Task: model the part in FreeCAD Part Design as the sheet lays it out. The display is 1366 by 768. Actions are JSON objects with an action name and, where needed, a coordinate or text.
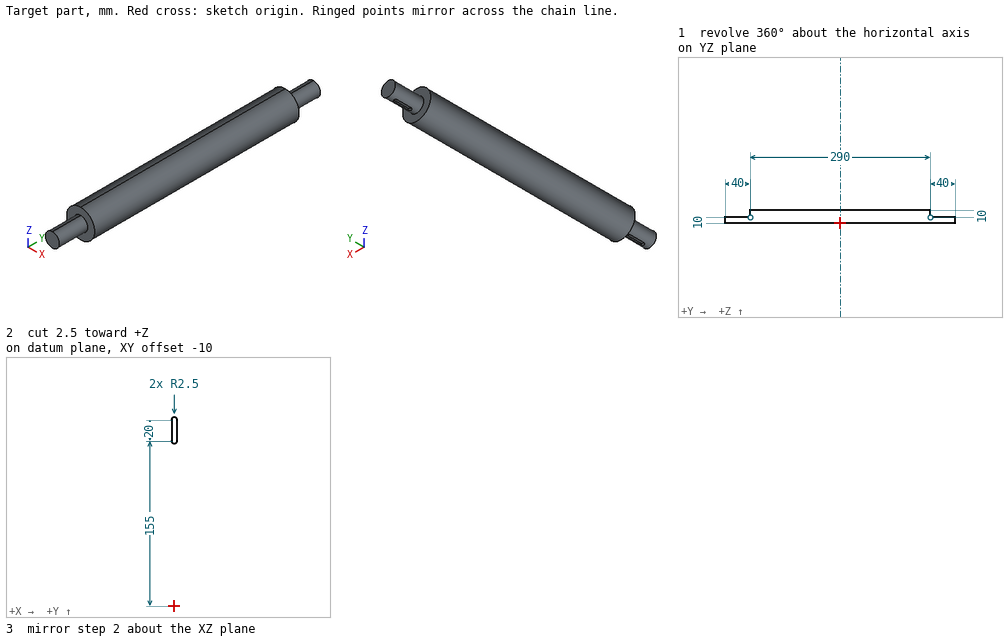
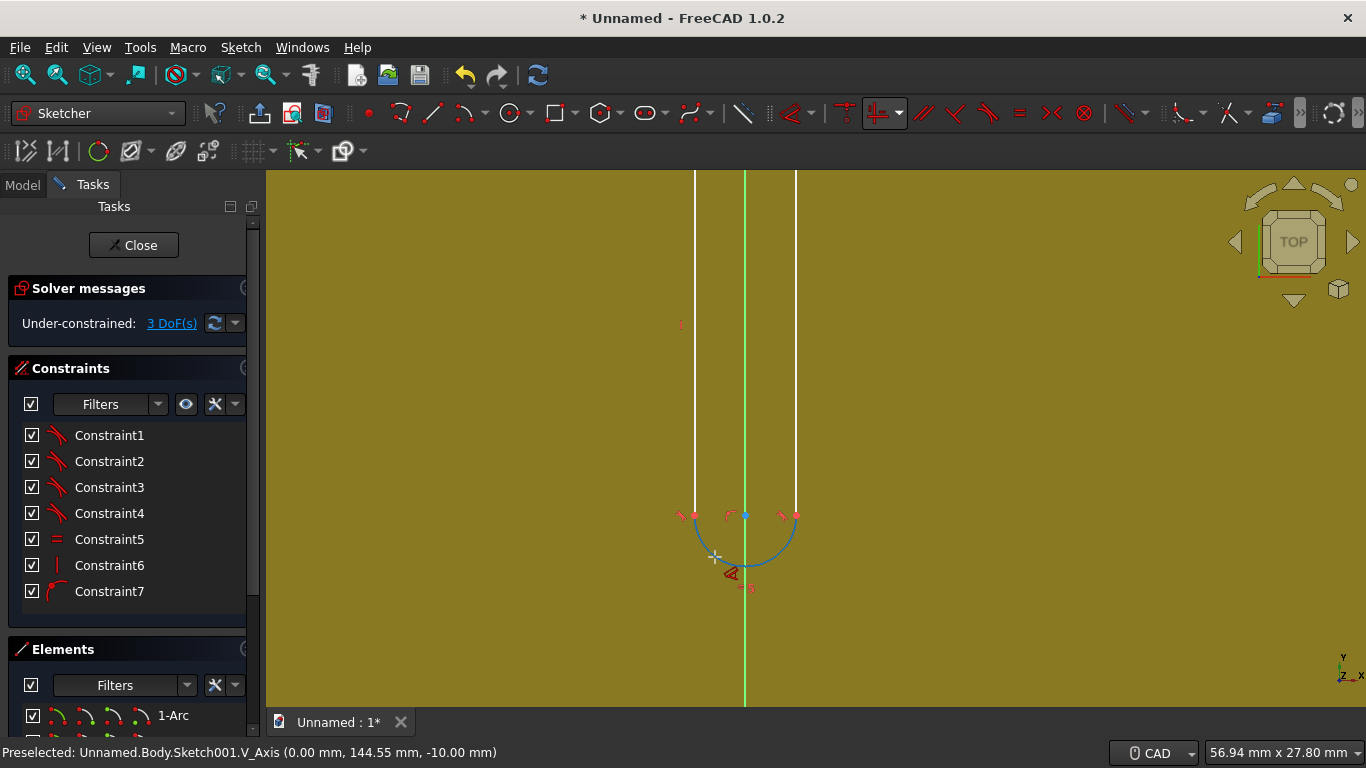
{"action": "left_click", "coordinate": [716, 557]}
{"action": "left_click", "coordinate": [697, 583]}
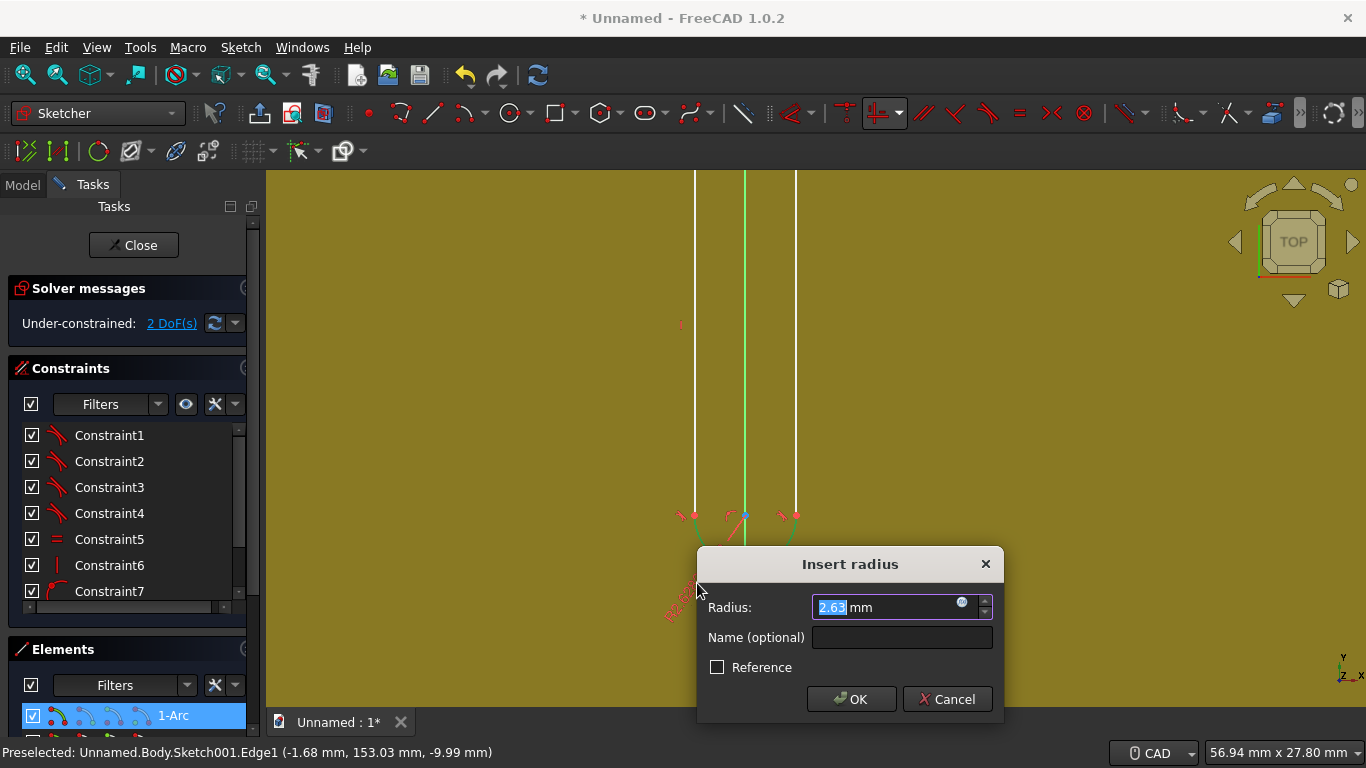
{"action": "type", "text": "2.5"}
{"action": "key", "text": "Return"}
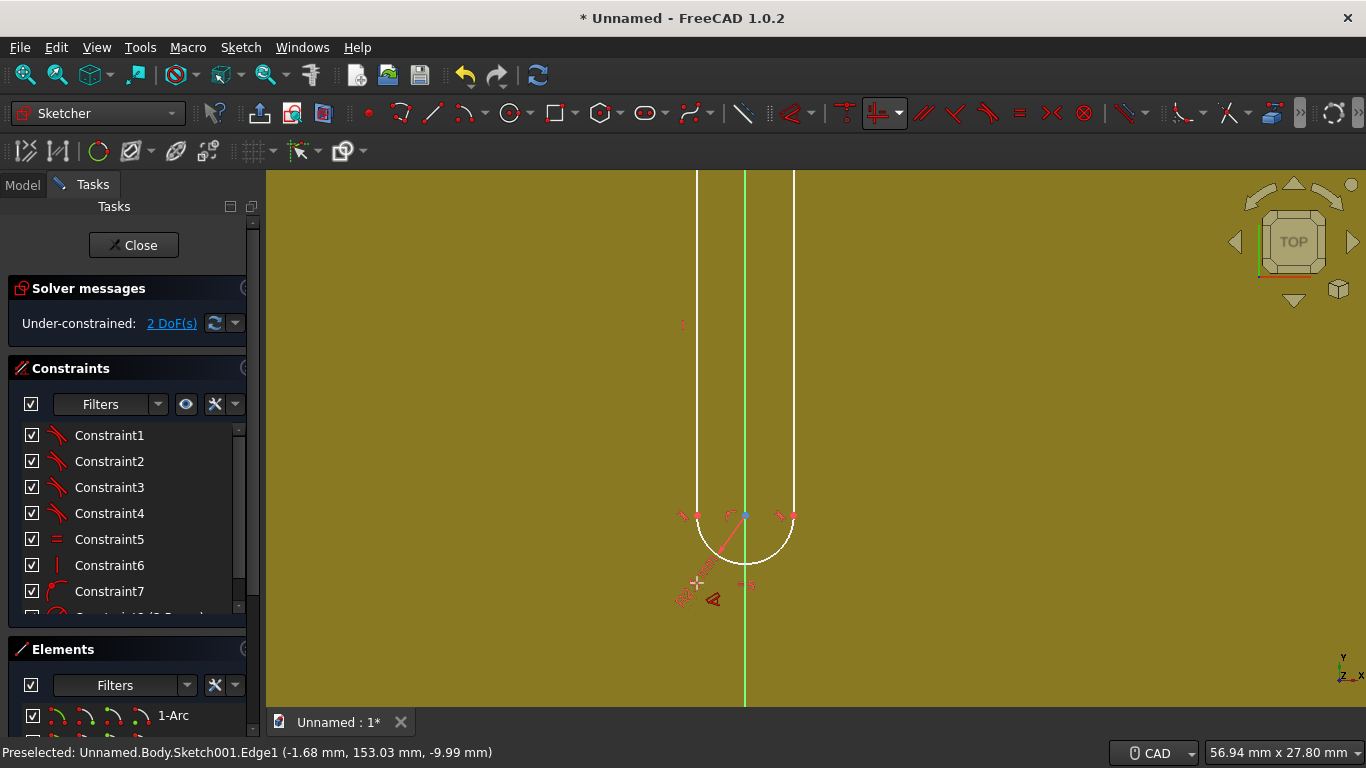
{"action": "left_click", "coordinate": [697, 401]}
{"action": "left_click", "coordinate": [663, 357]}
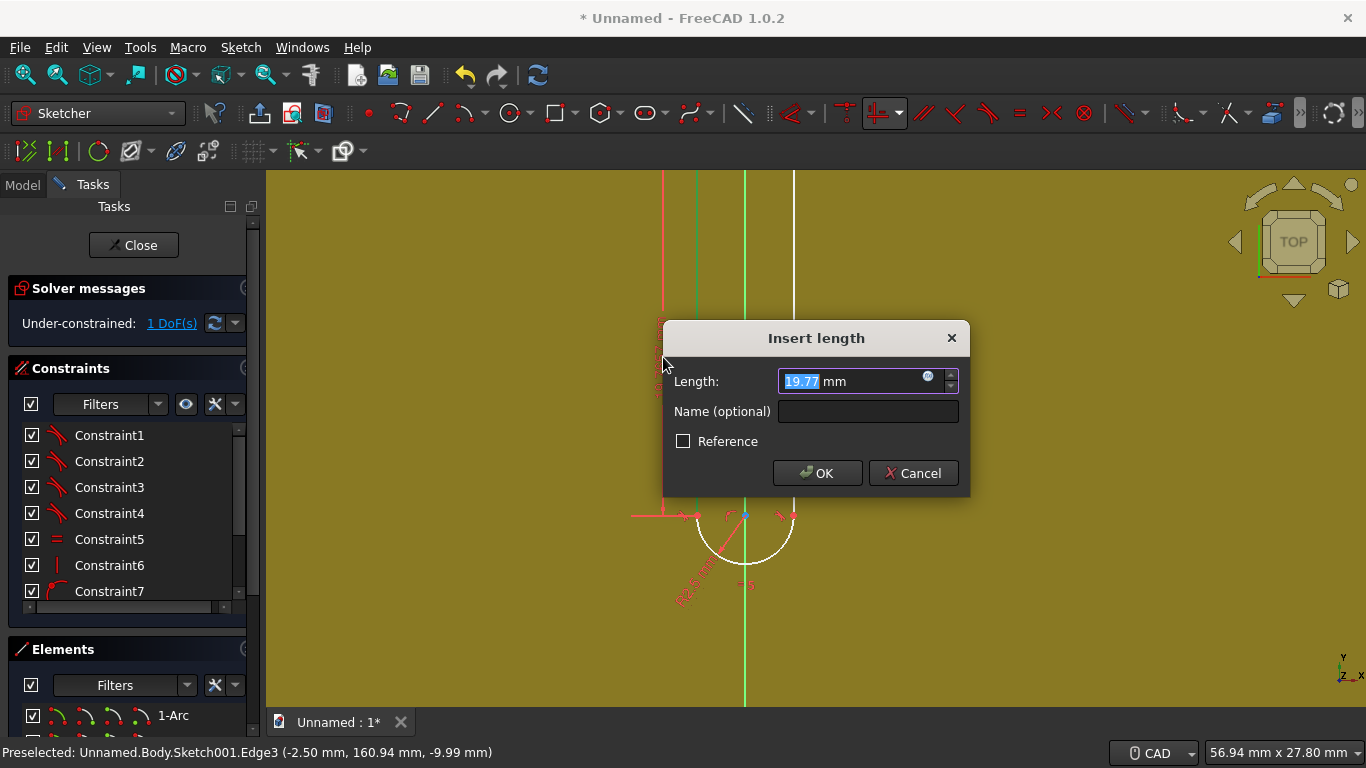
{"action": "type", "text": "20"}
{"action": "key", "text": "Return"}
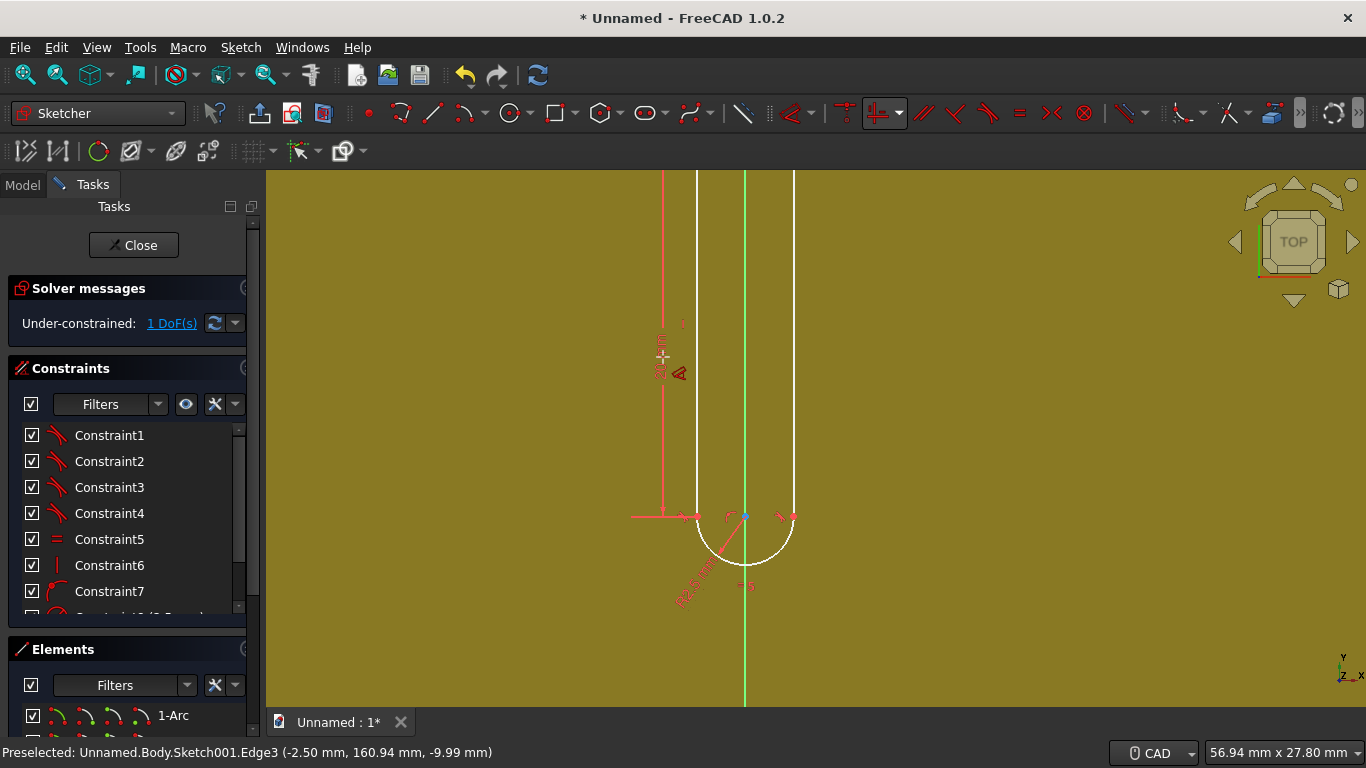
{"action": "left_click", "coordinate": [697, 517]}
{"action": "left_click", "coordinate": [663, 560]}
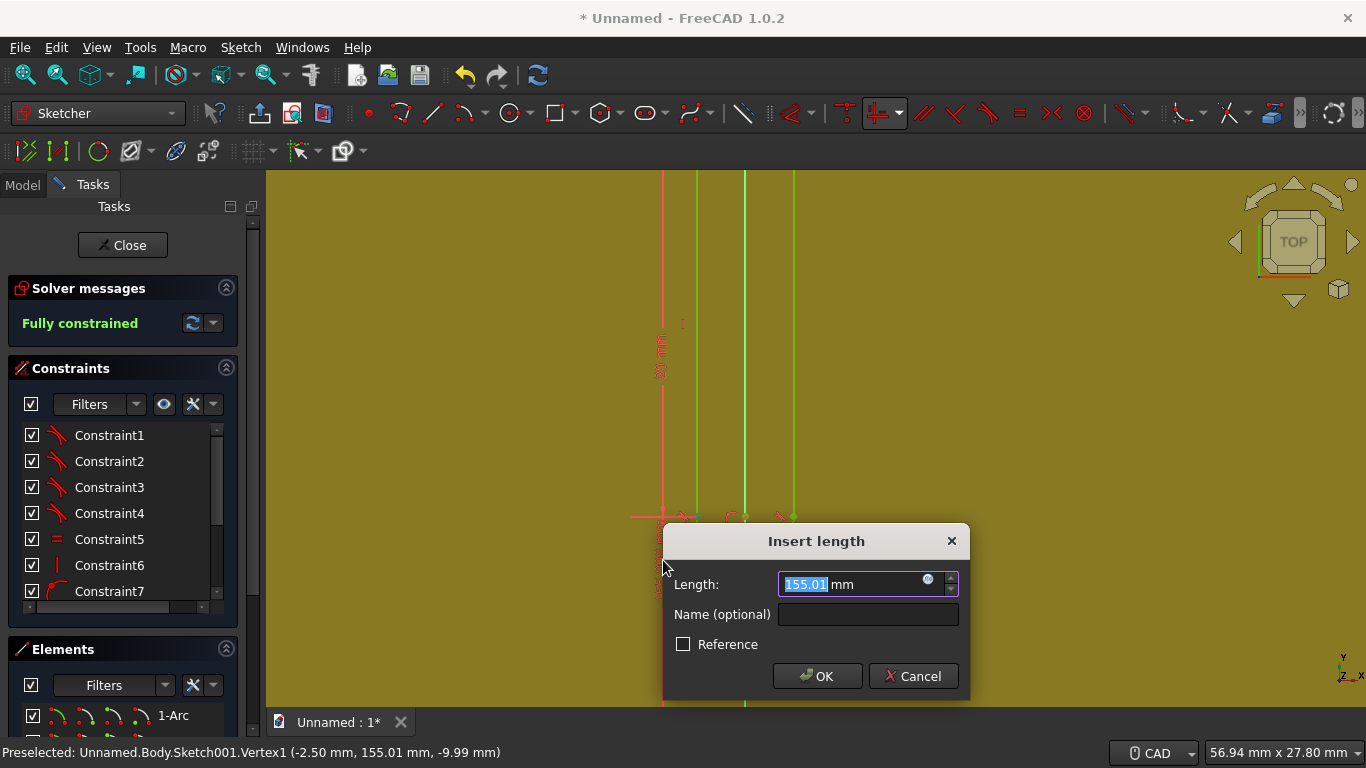
{"action": "type", "text": "155"}
{"action": "key", "text": "Return"}
{"action": "key", "text": "Escape"}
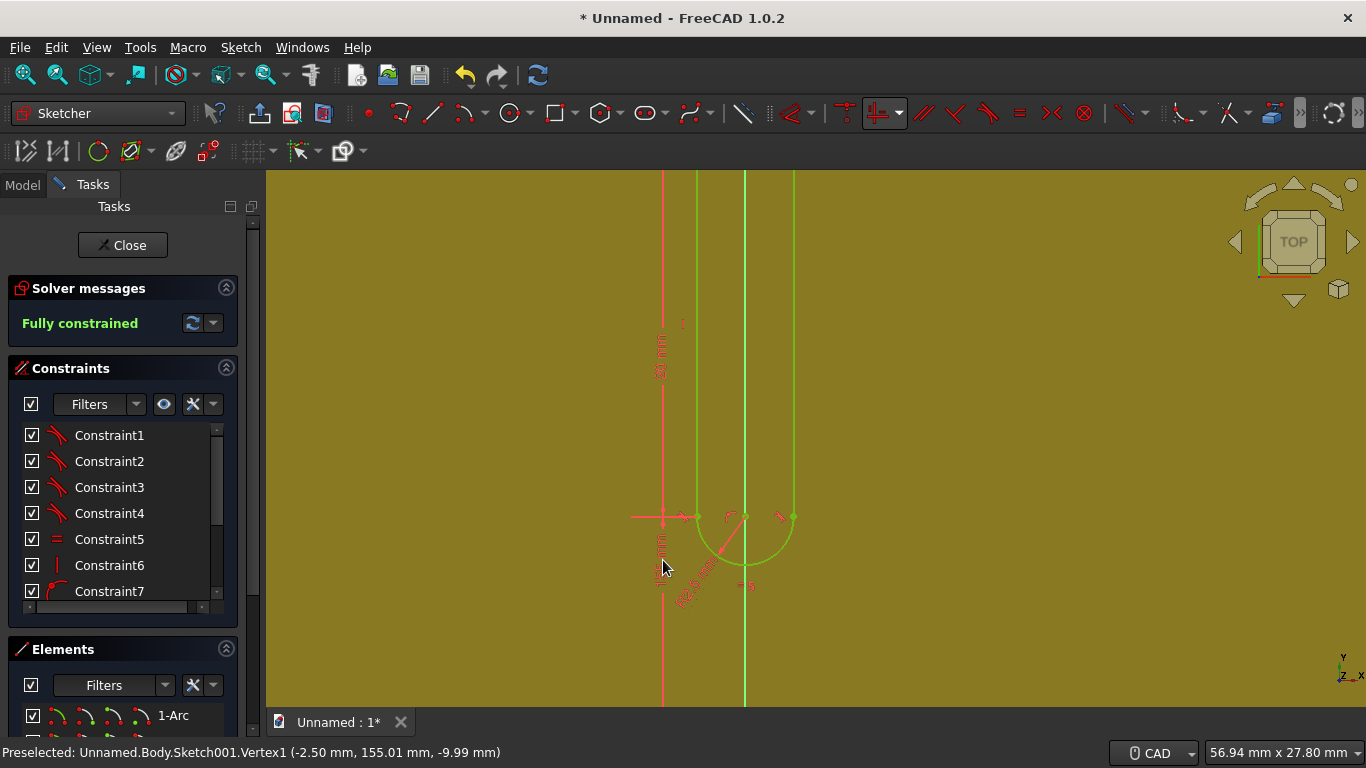
{"action": "left_click", "coordinate": [123, 245]}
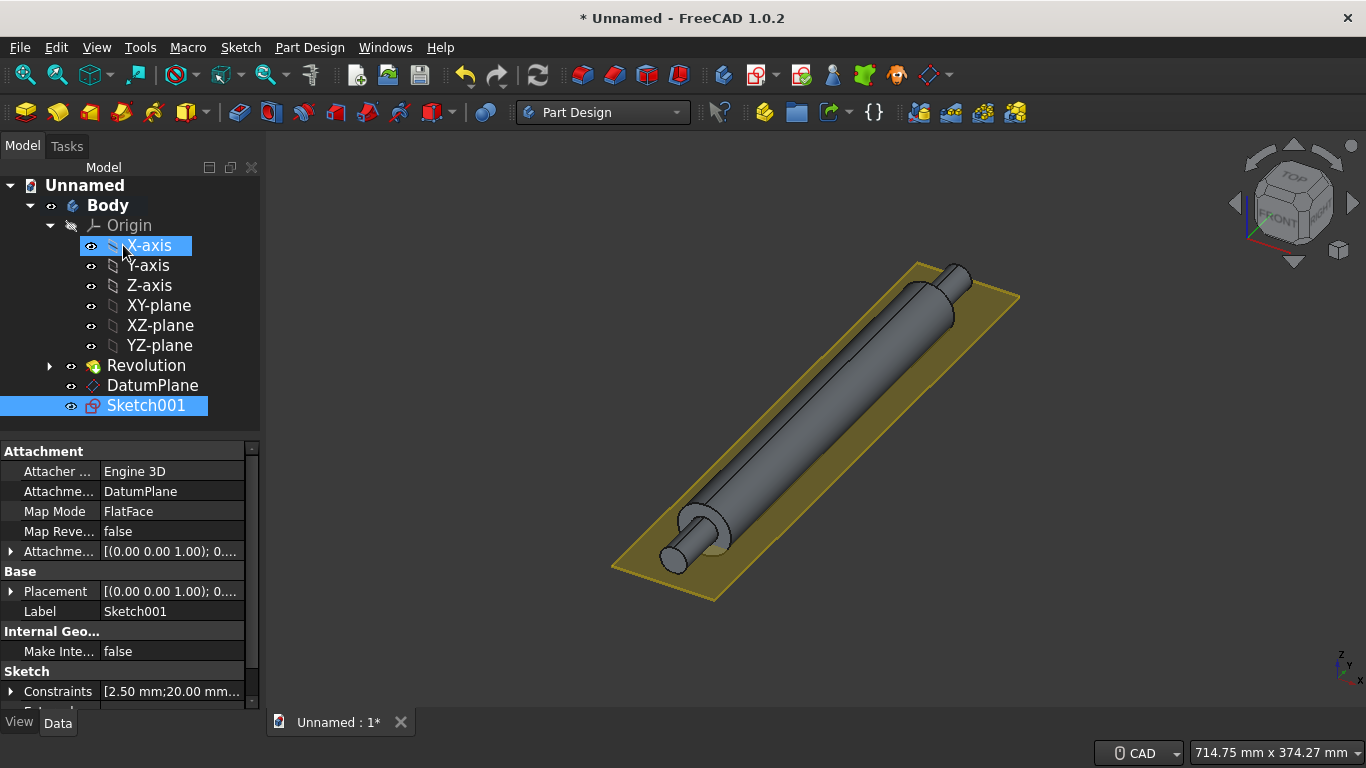
{"action": "left_click", "coordinate": [240, 112]}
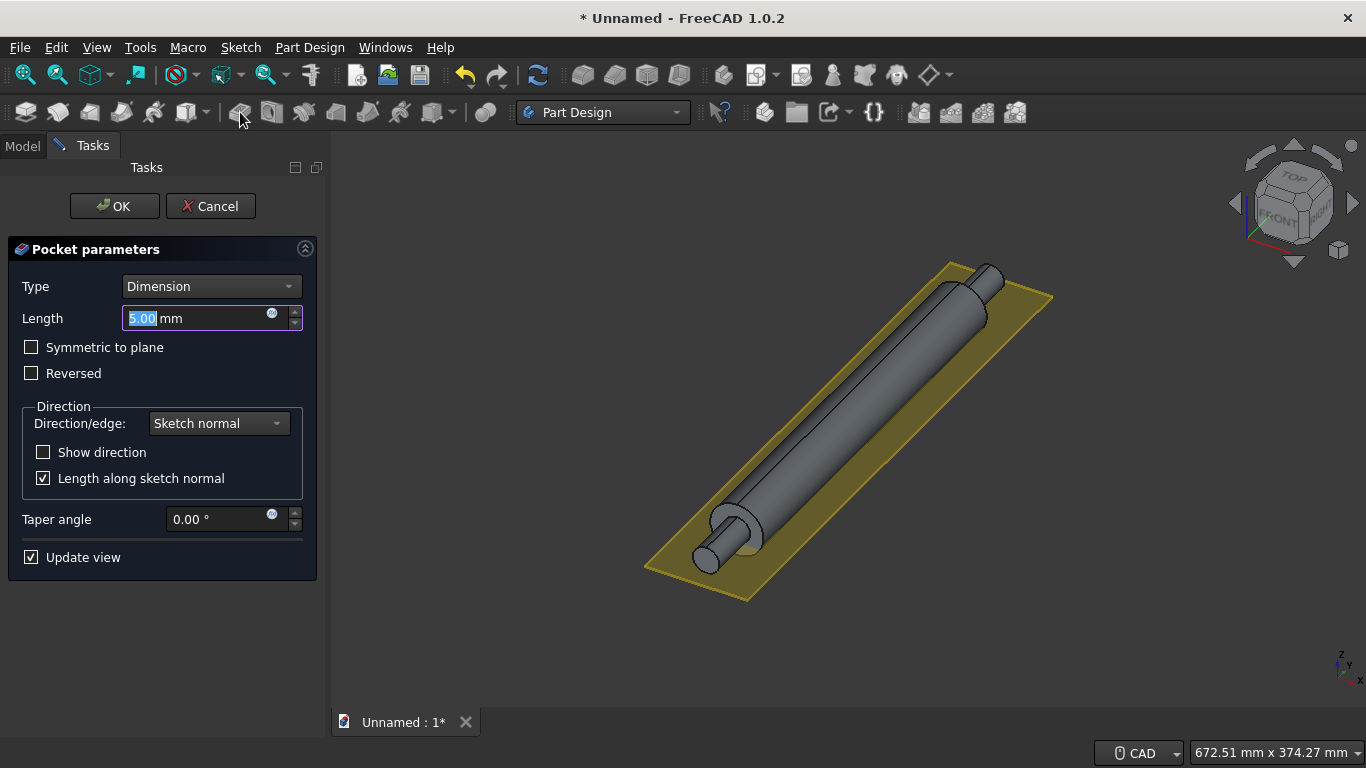
{"action": "type", "text": "2.5"}
{"action": "key", "text": "Tab"}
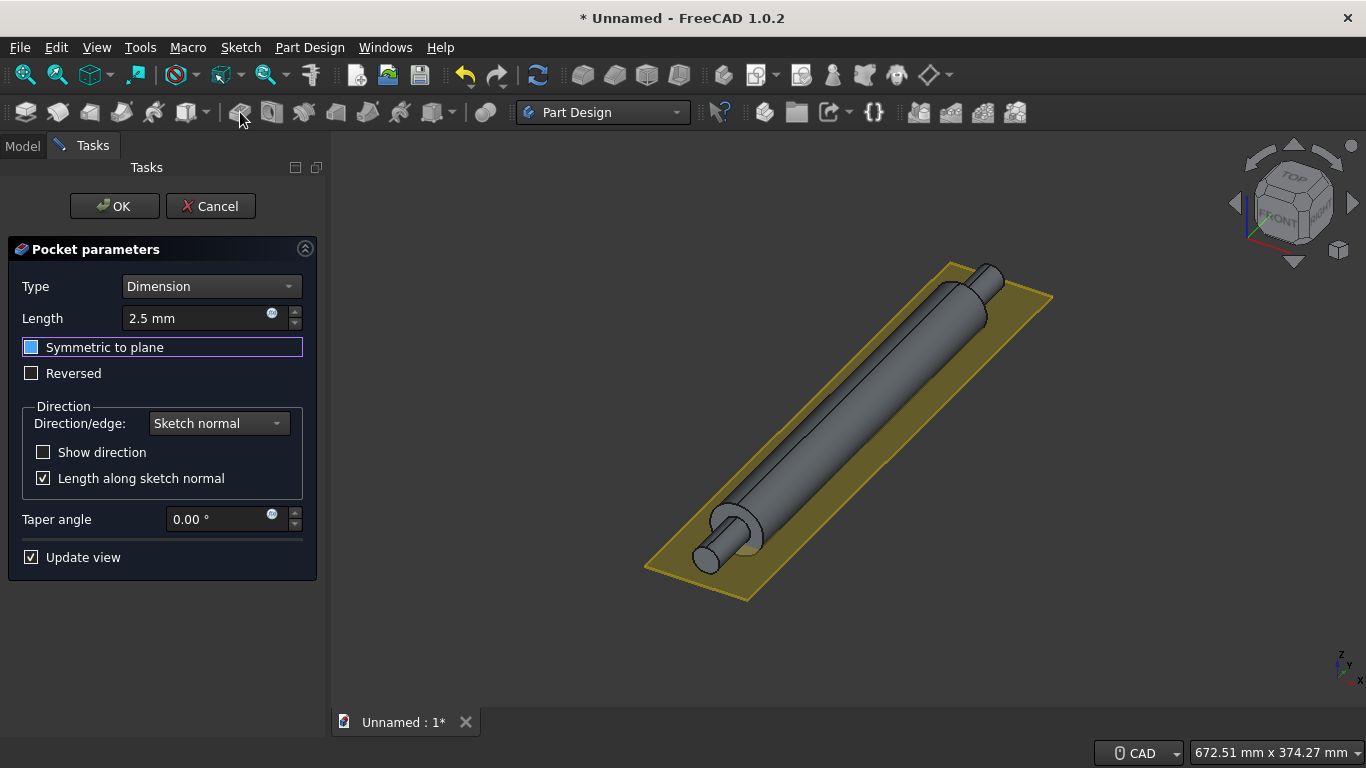
{"action": "left_click", "coordinate": [30, 373]}